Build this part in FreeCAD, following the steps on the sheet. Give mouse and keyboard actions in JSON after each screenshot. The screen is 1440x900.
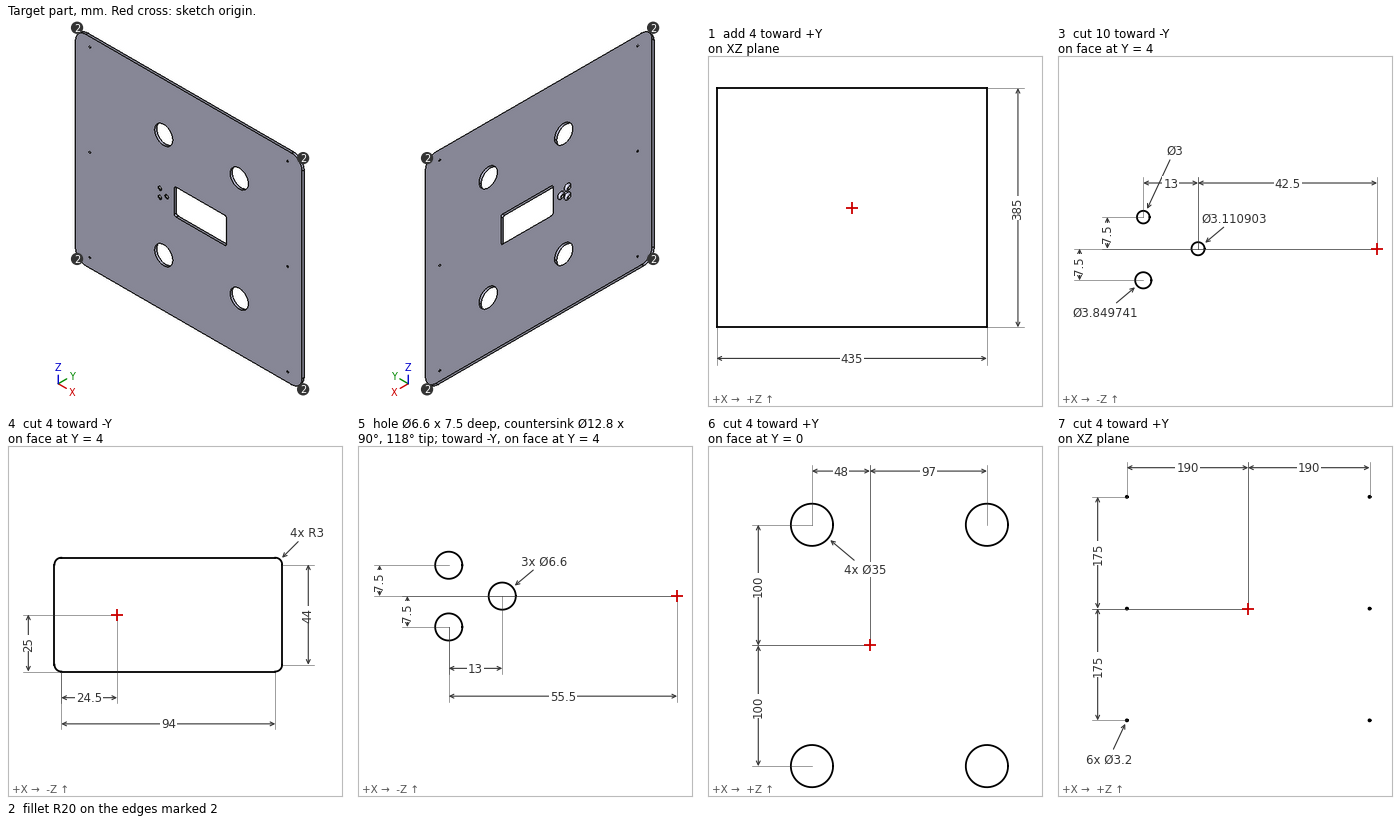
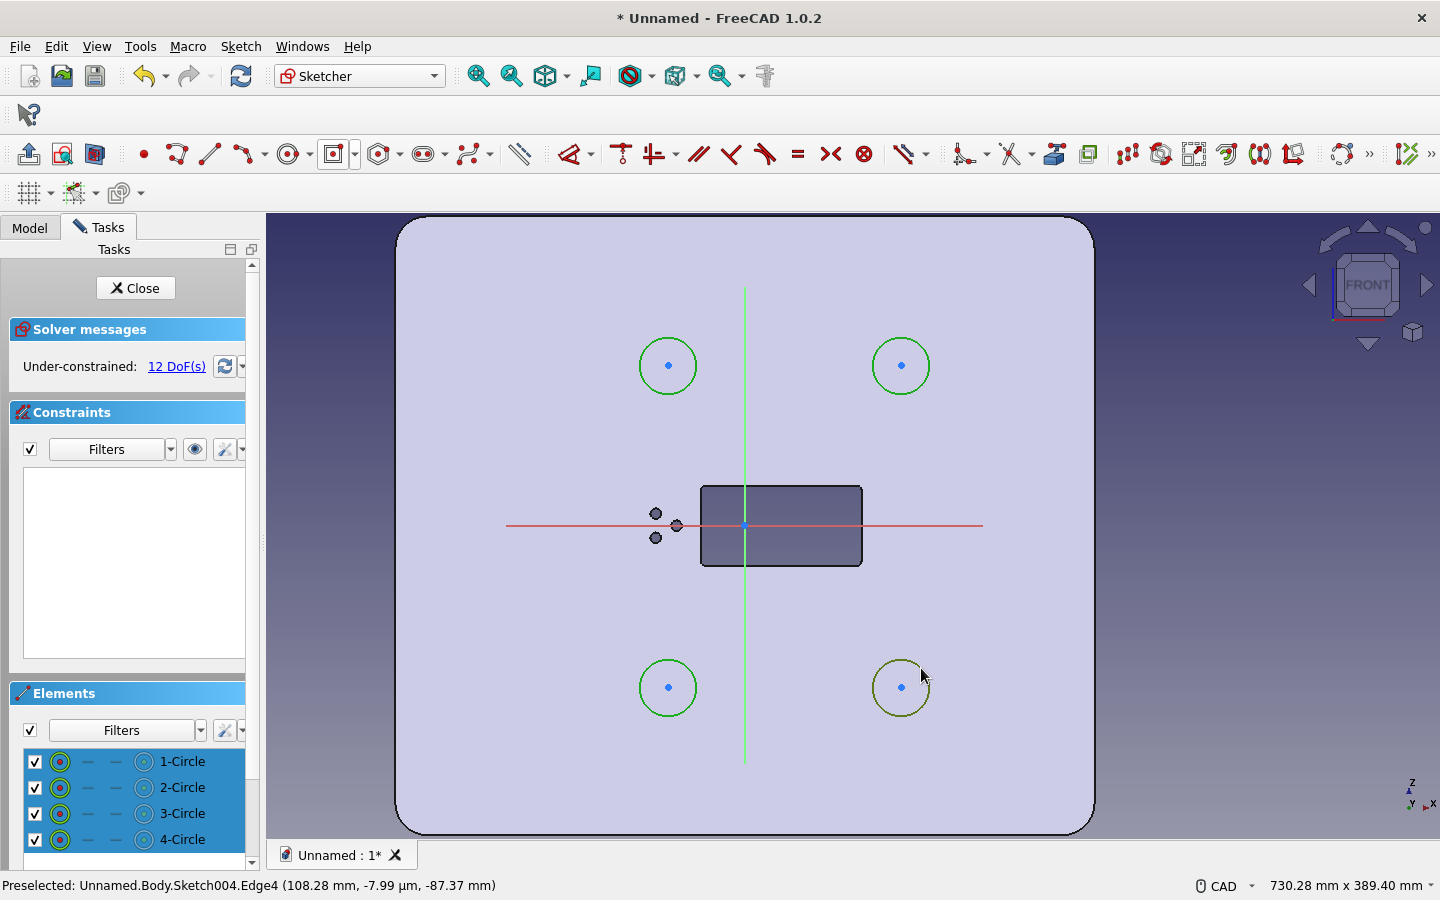
{"action": "left_click", "coordinate": [798, 154]}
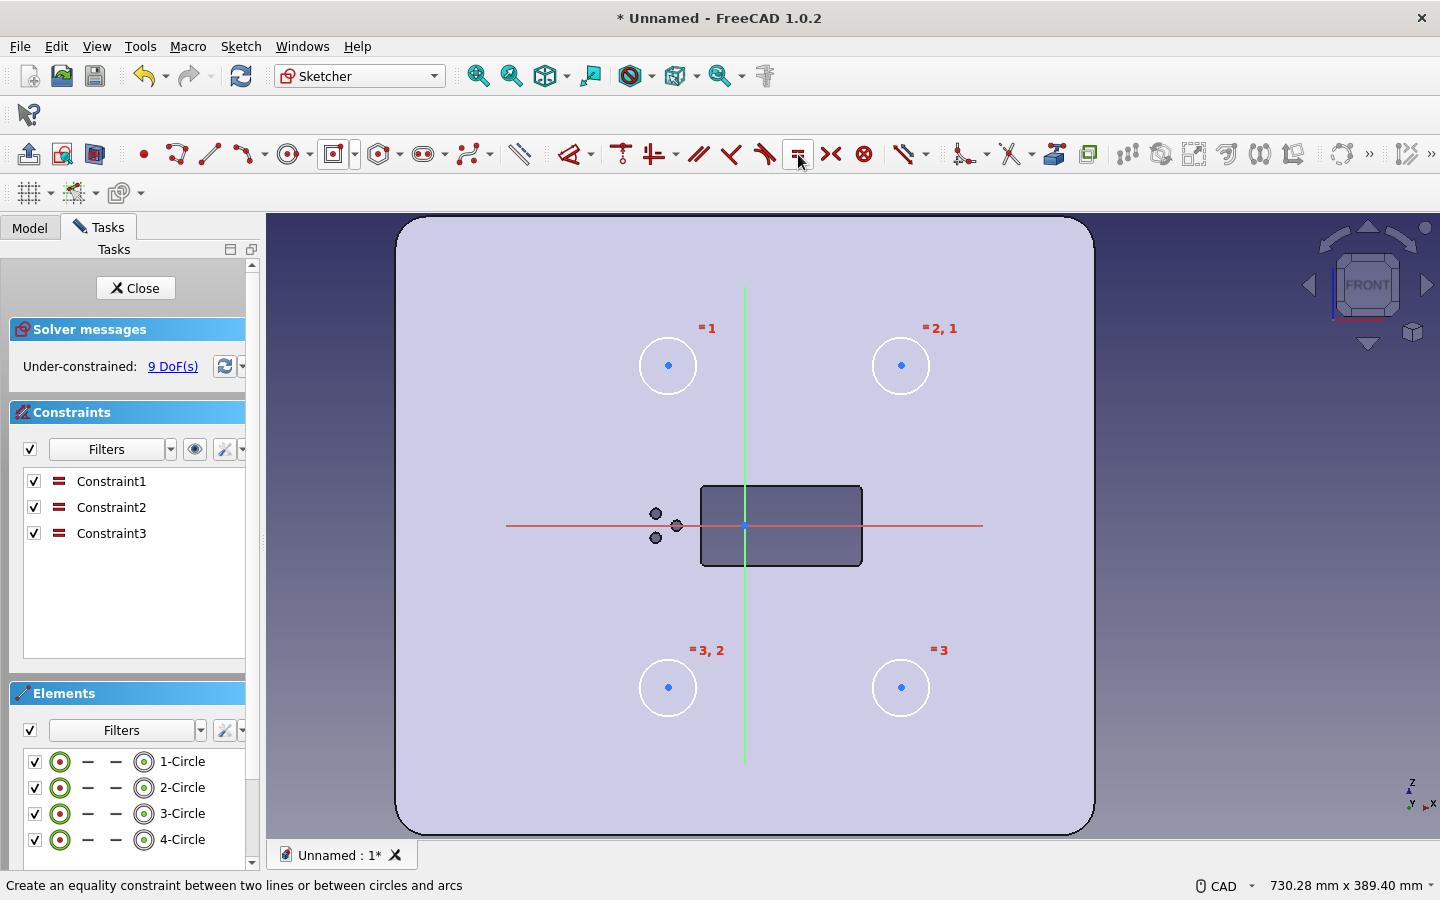
{"action": "left_click", "coordinate": [668, 366]}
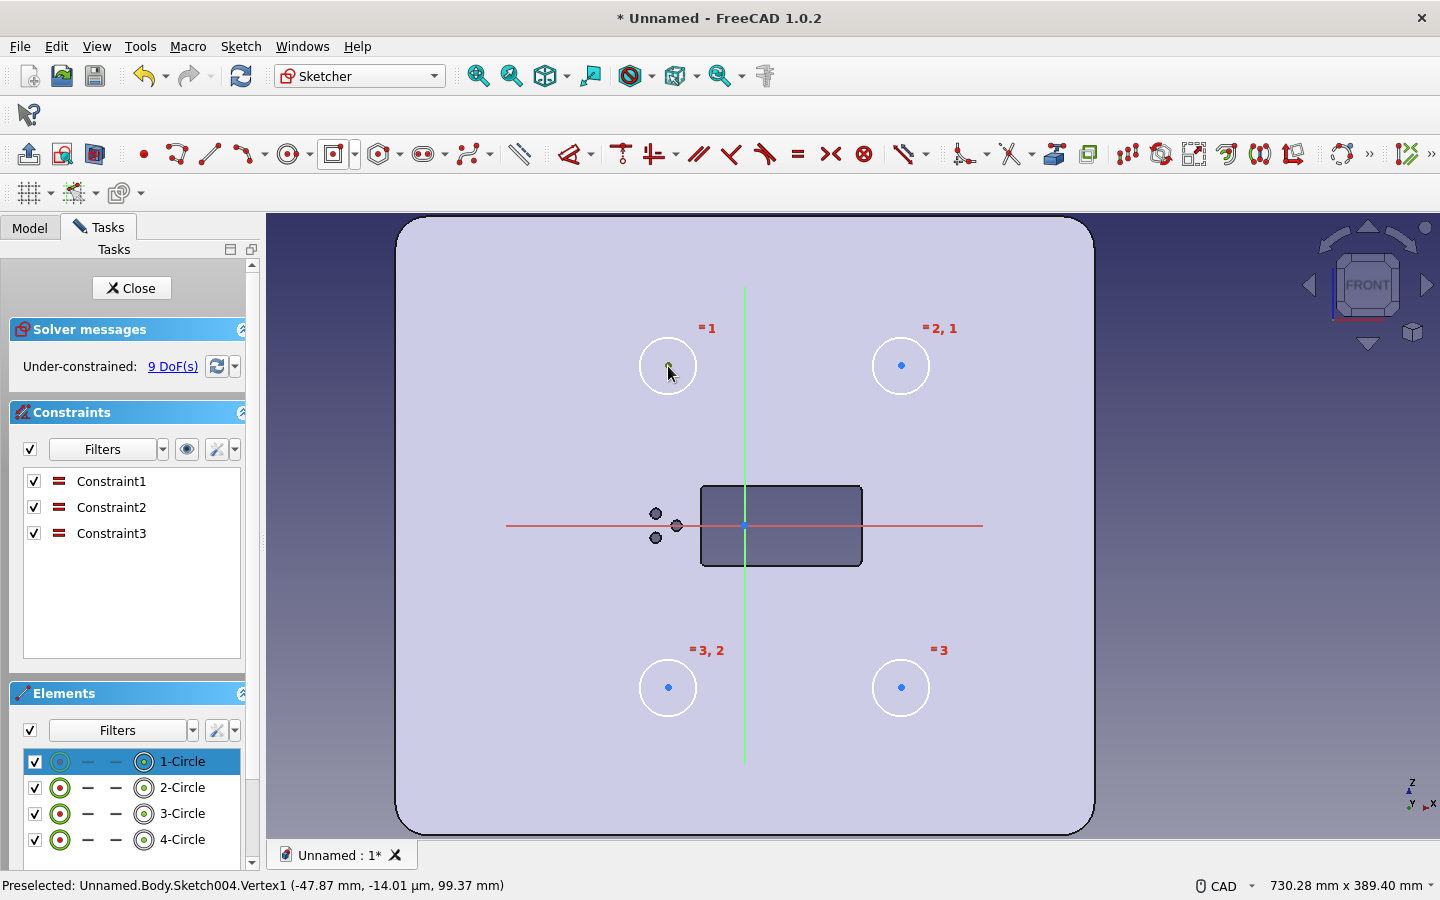
{"action": "left_click", "coordinate": [901, 366]}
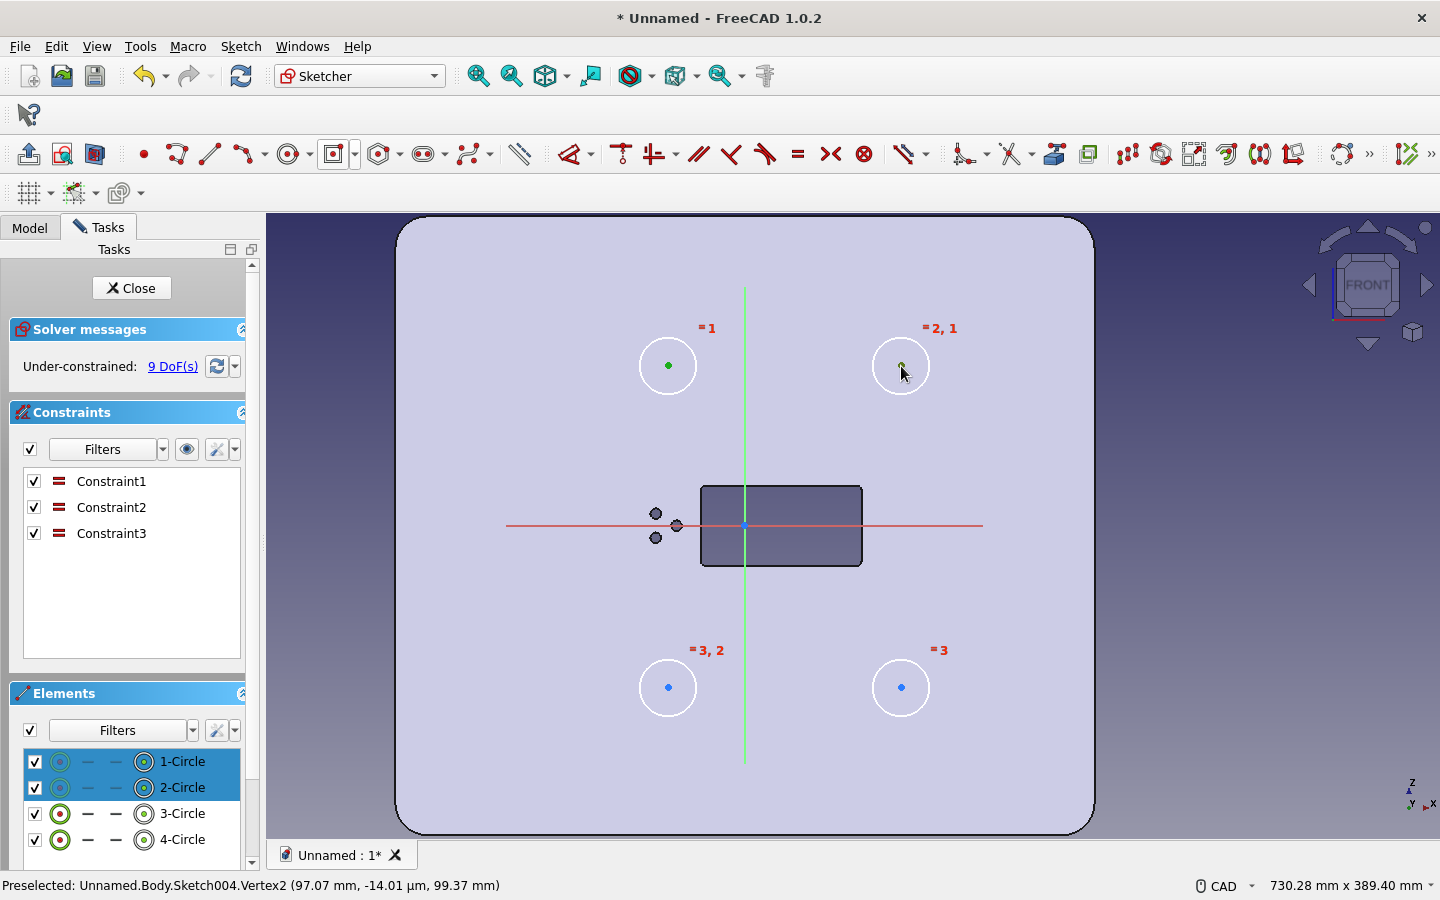
{"action": "left_click", "coordinate": [676, 154]}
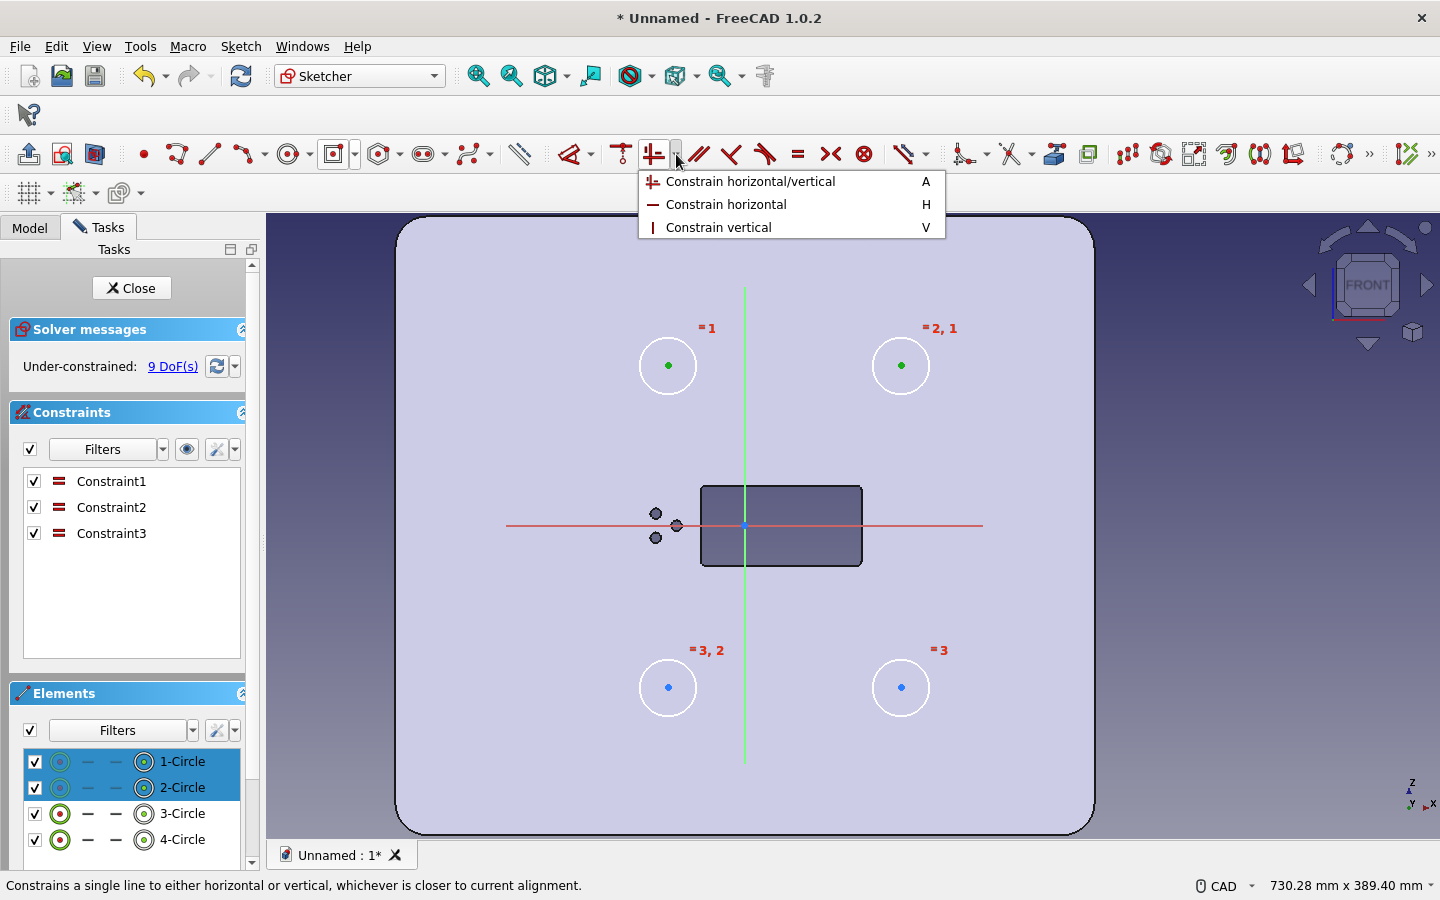
{"action": "left_click", "coordinate": [792, 204]}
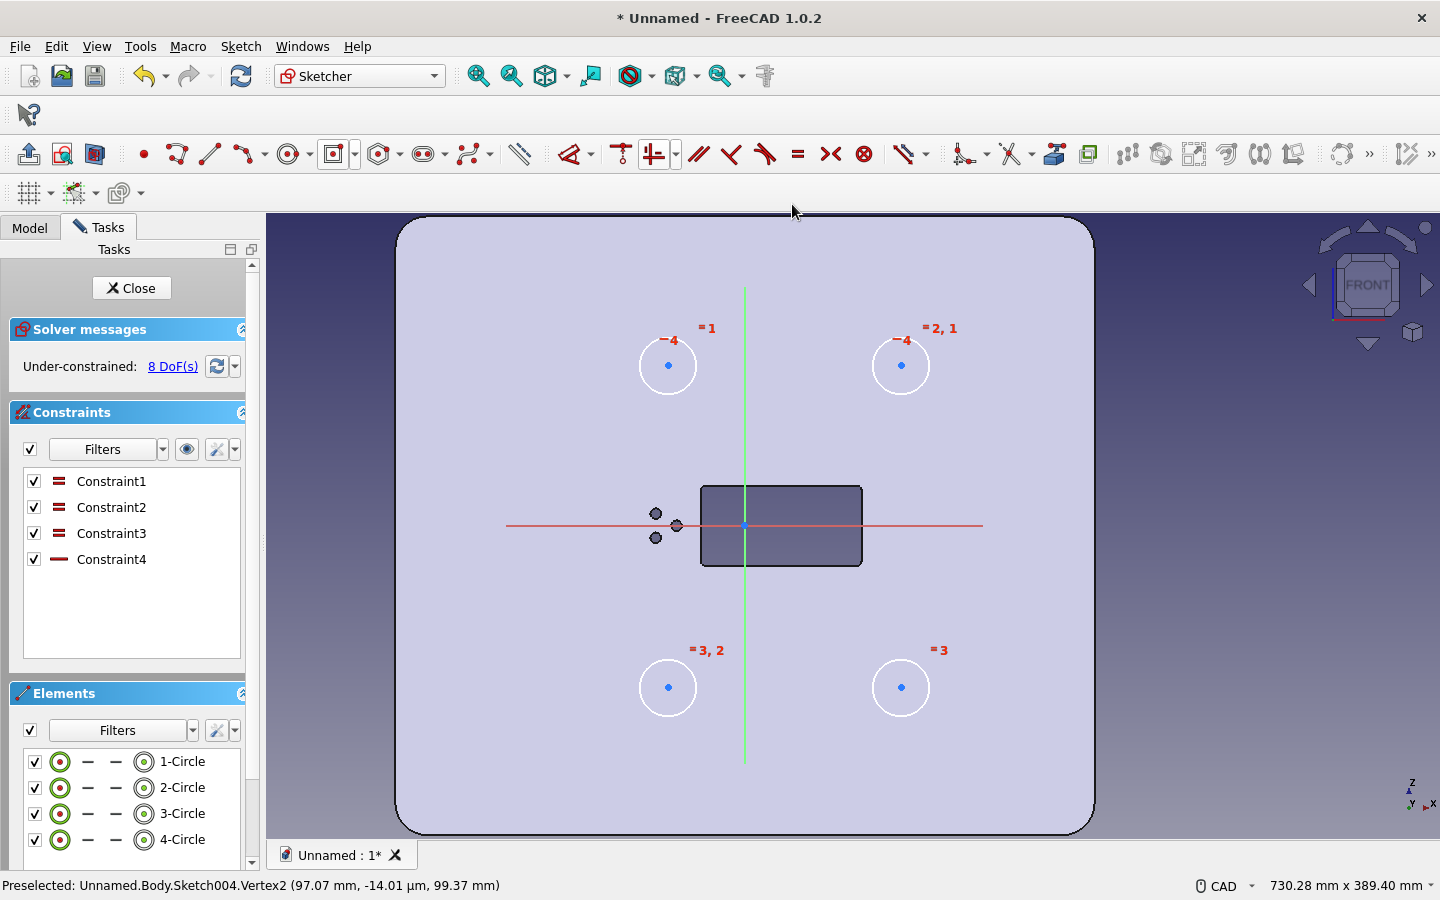
{"action": "left_click", "coordinate": [668, 366]}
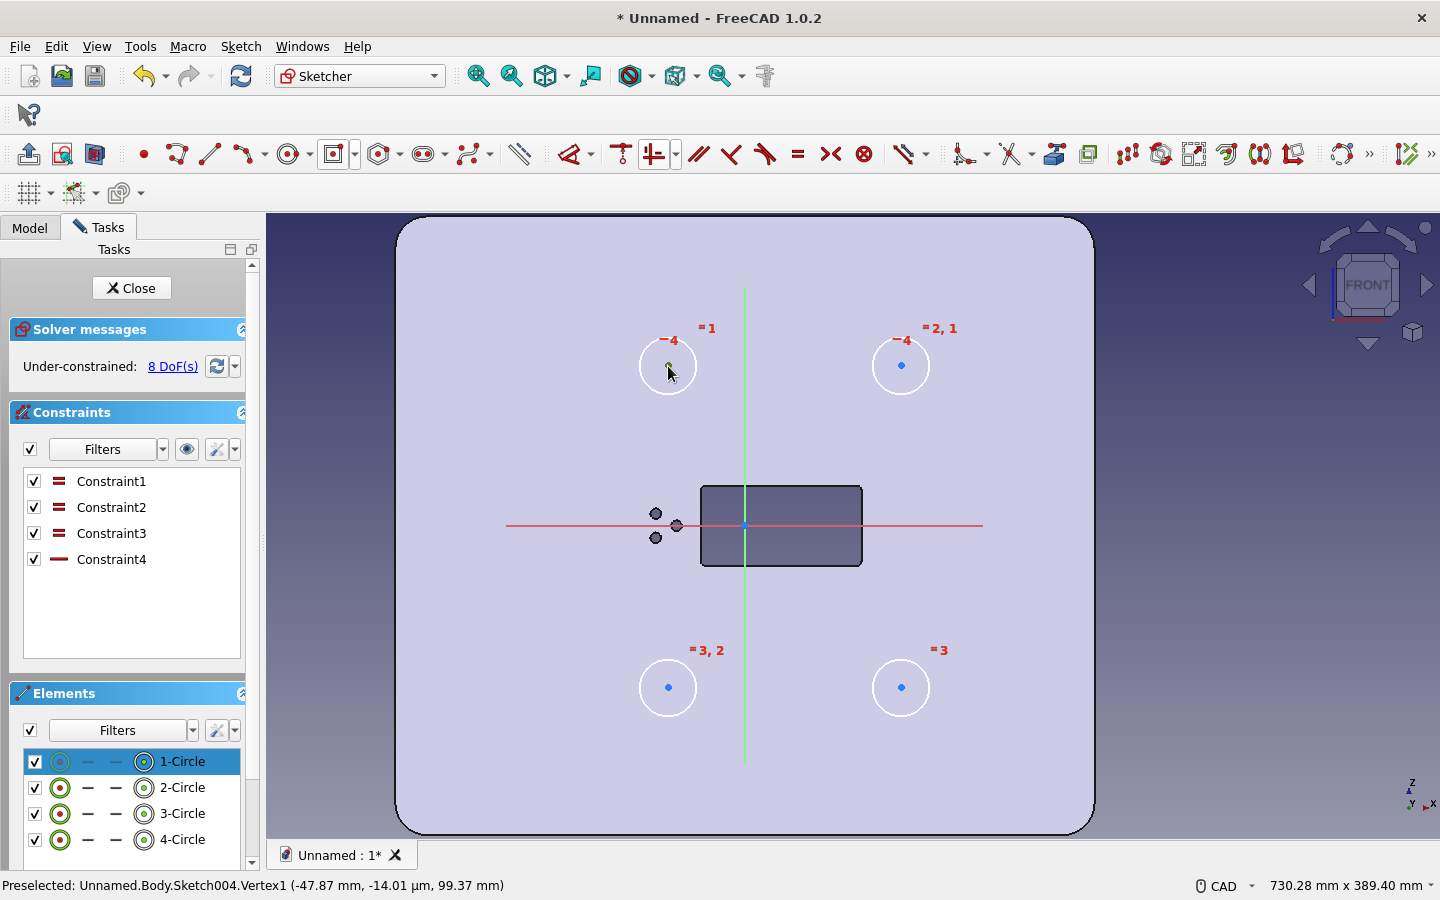
{"action": "left_click", "coordinate": [668, 688]}